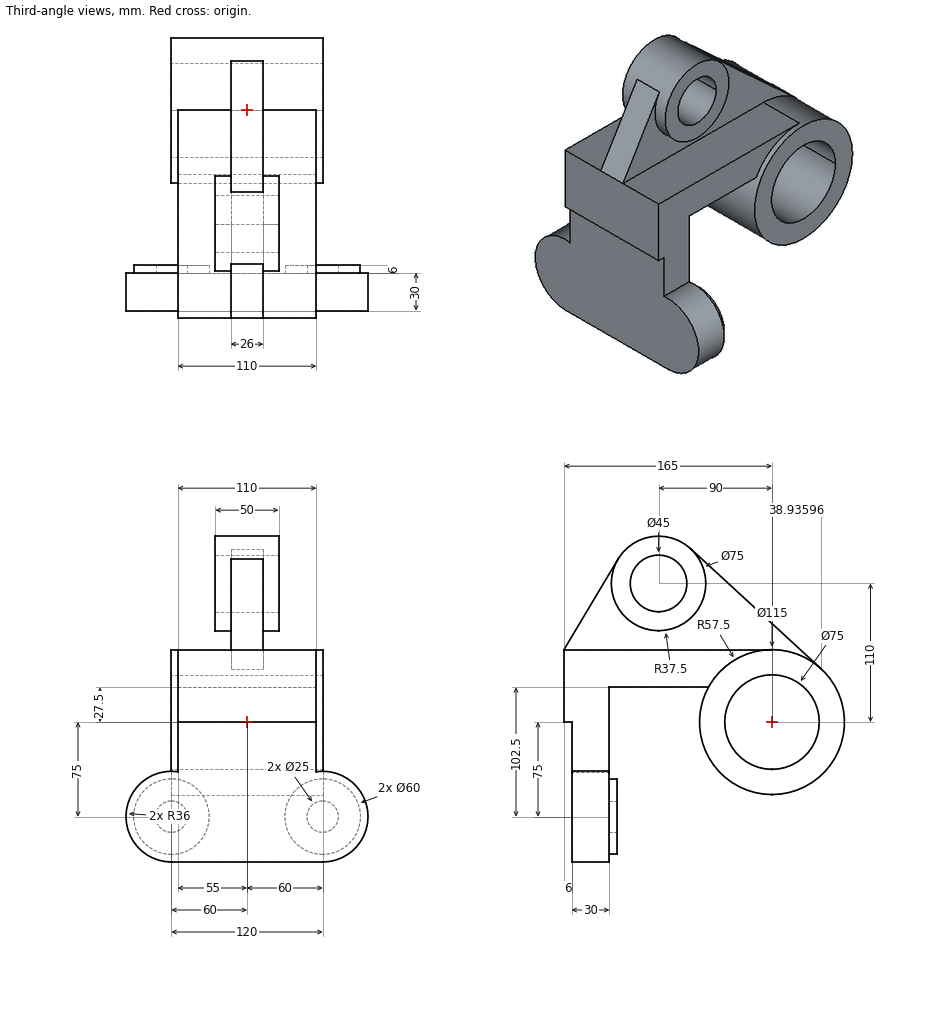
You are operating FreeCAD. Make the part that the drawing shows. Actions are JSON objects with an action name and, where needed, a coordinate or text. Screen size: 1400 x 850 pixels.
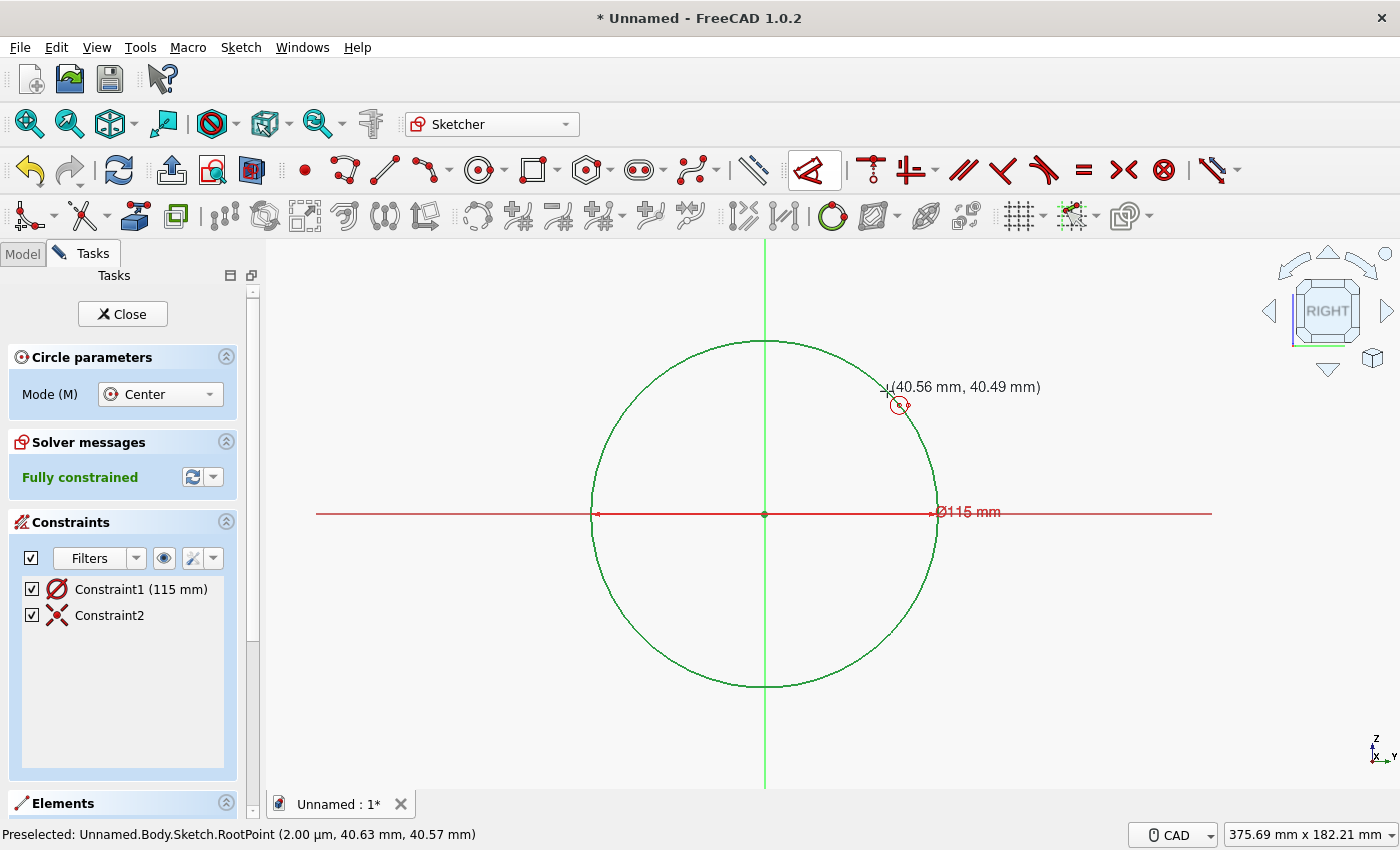
{"action": "left_click", "coordinate": [765, 514]}
{"action": "mouse_move", "coordinate": [845, 434]}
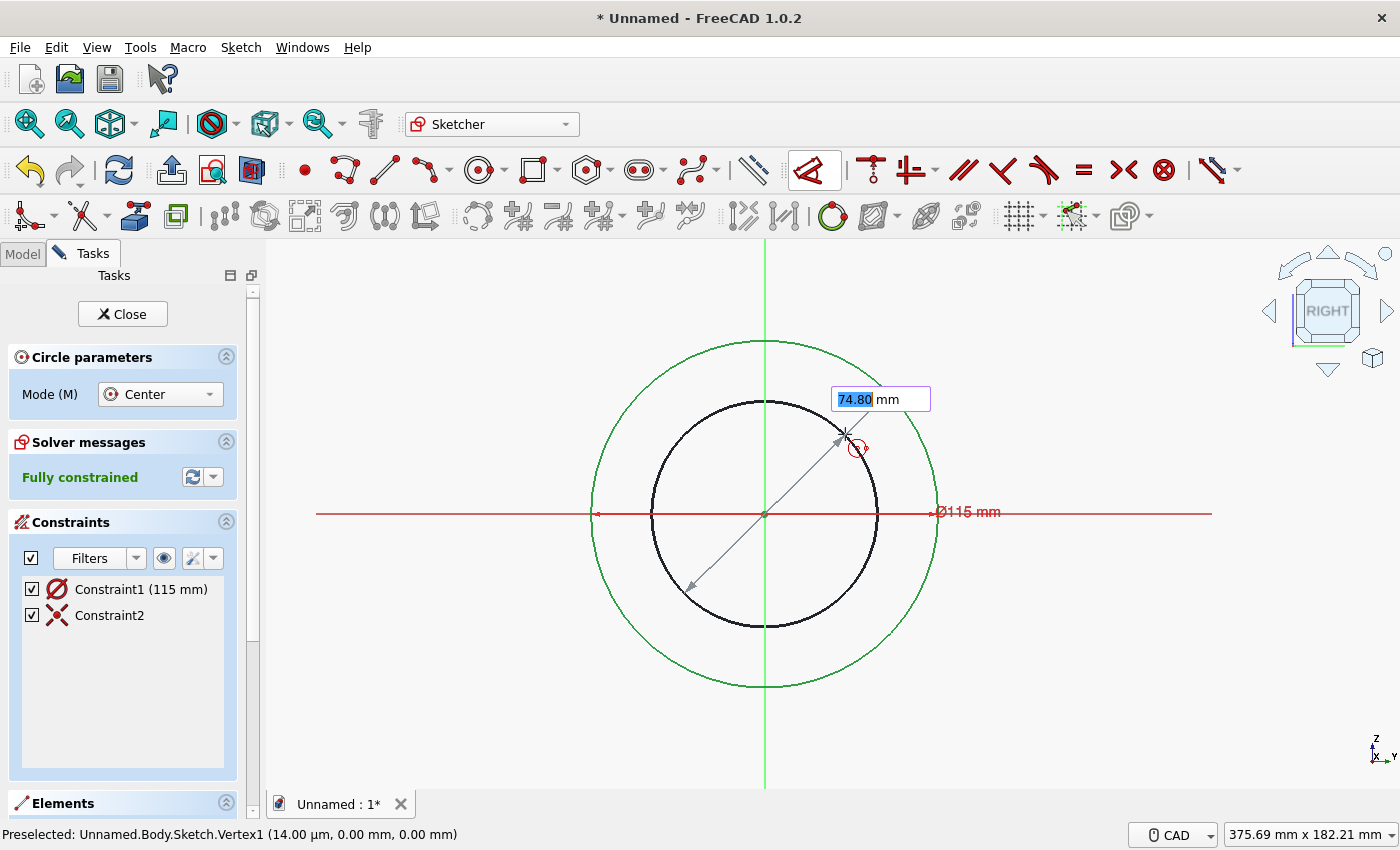
{"action": "type", "text": "75"}
{"action": "key", "text": "Return"}
{"action": "key", "text": "Escape"}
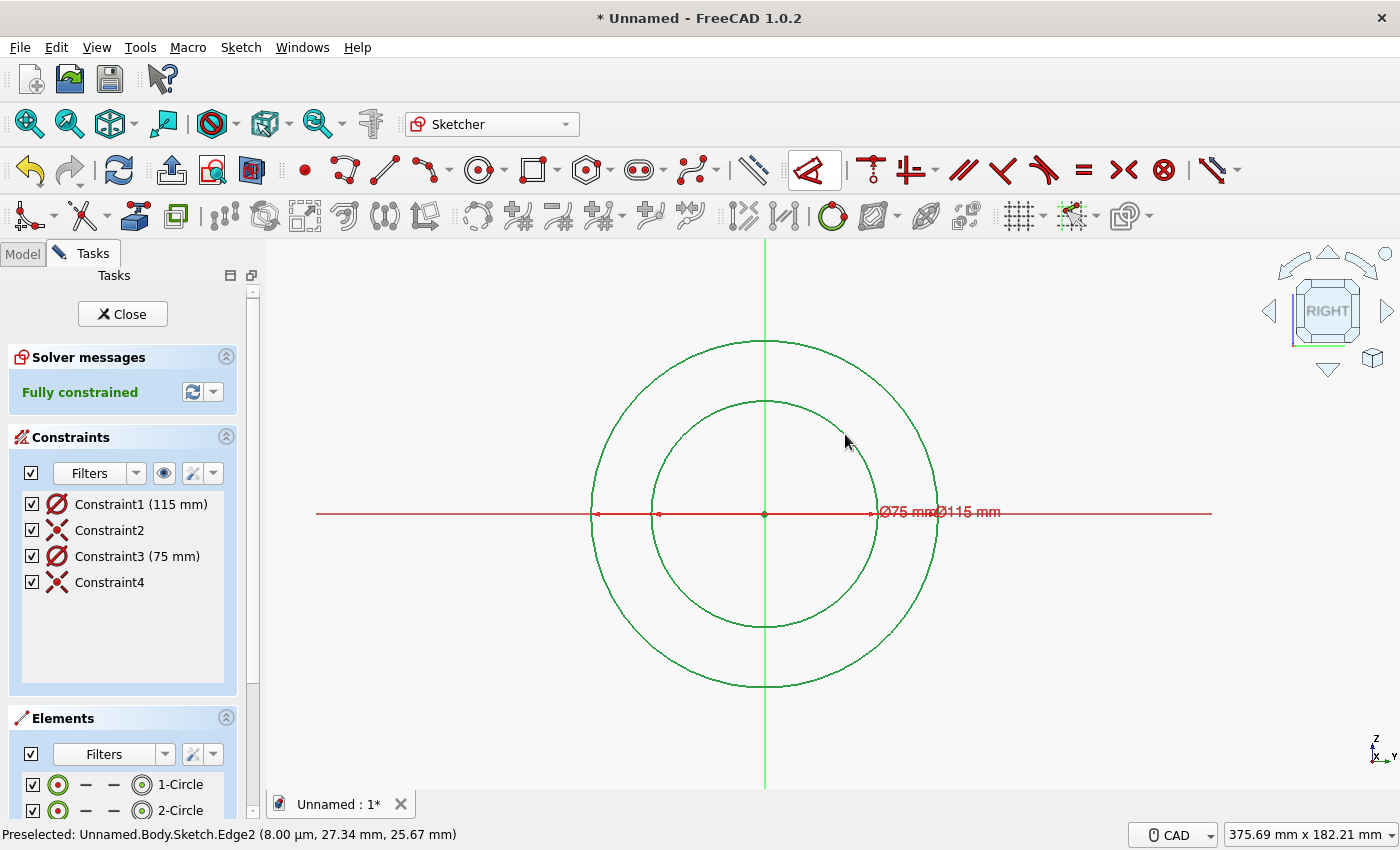
{"action": "left_click", "coordinate": [123, 314]}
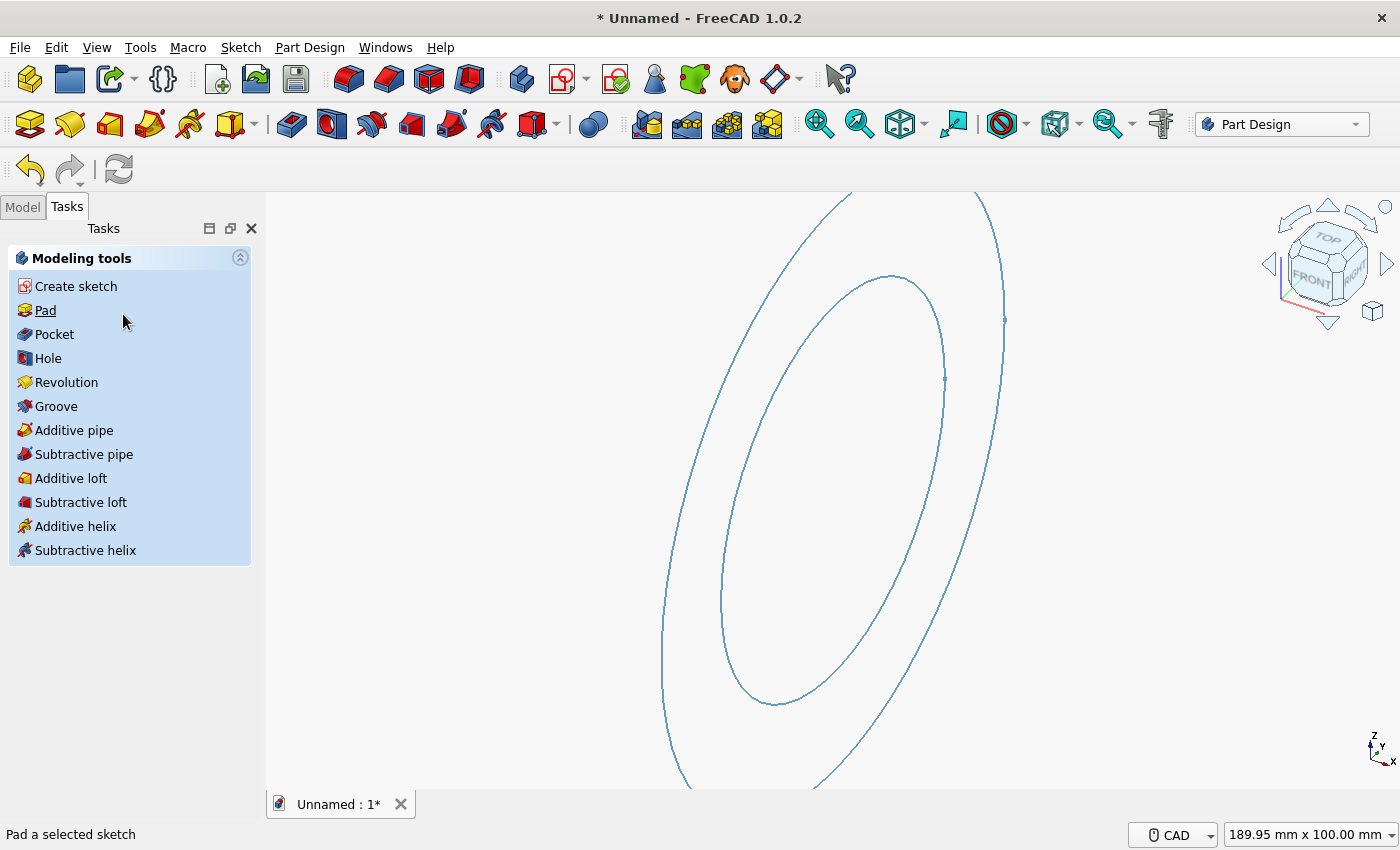
{"action": "left_click", "coordinate": [30, 124]}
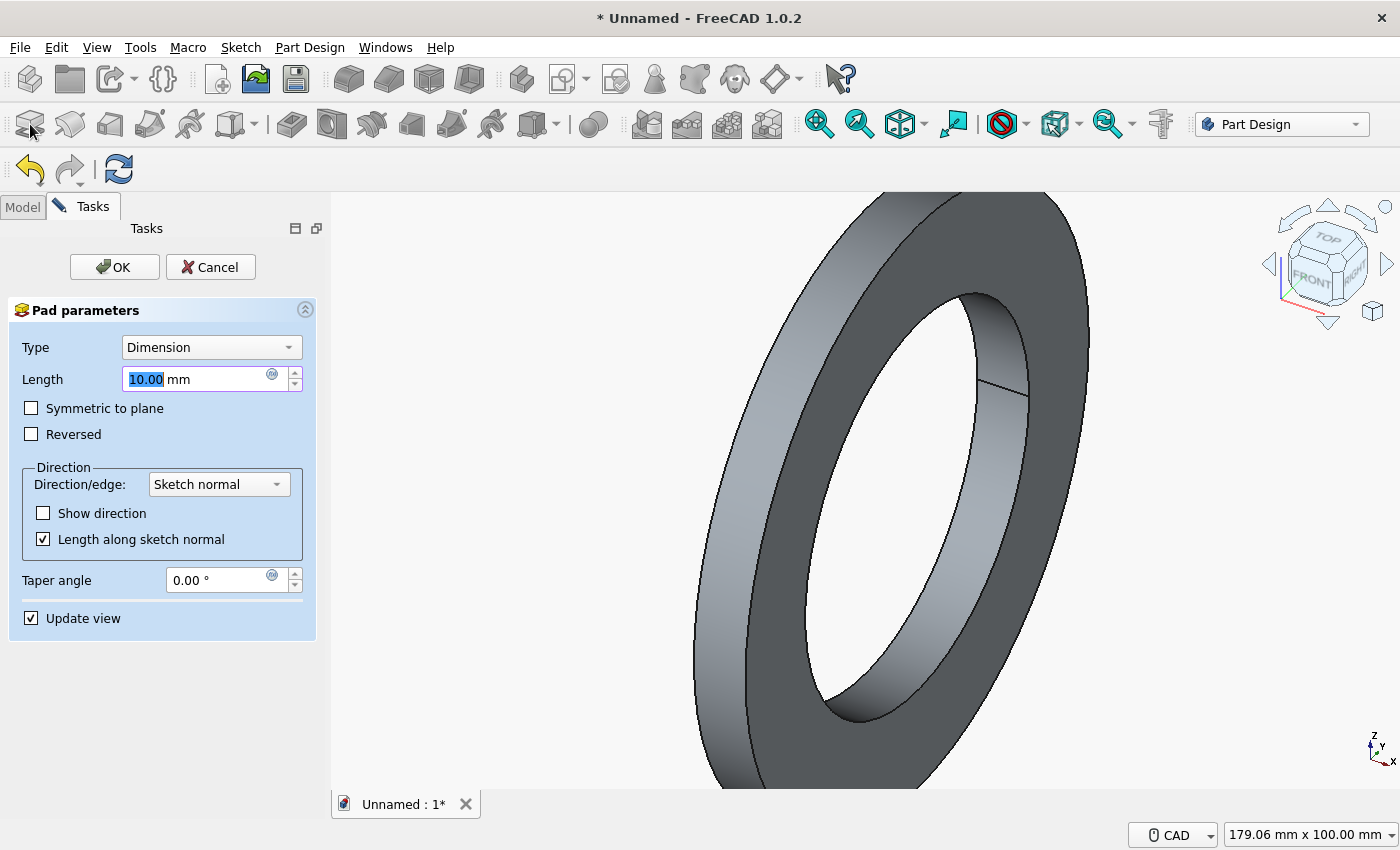
{"action": "type", "text": "120"}
{"action": "key", "text": "Tab"}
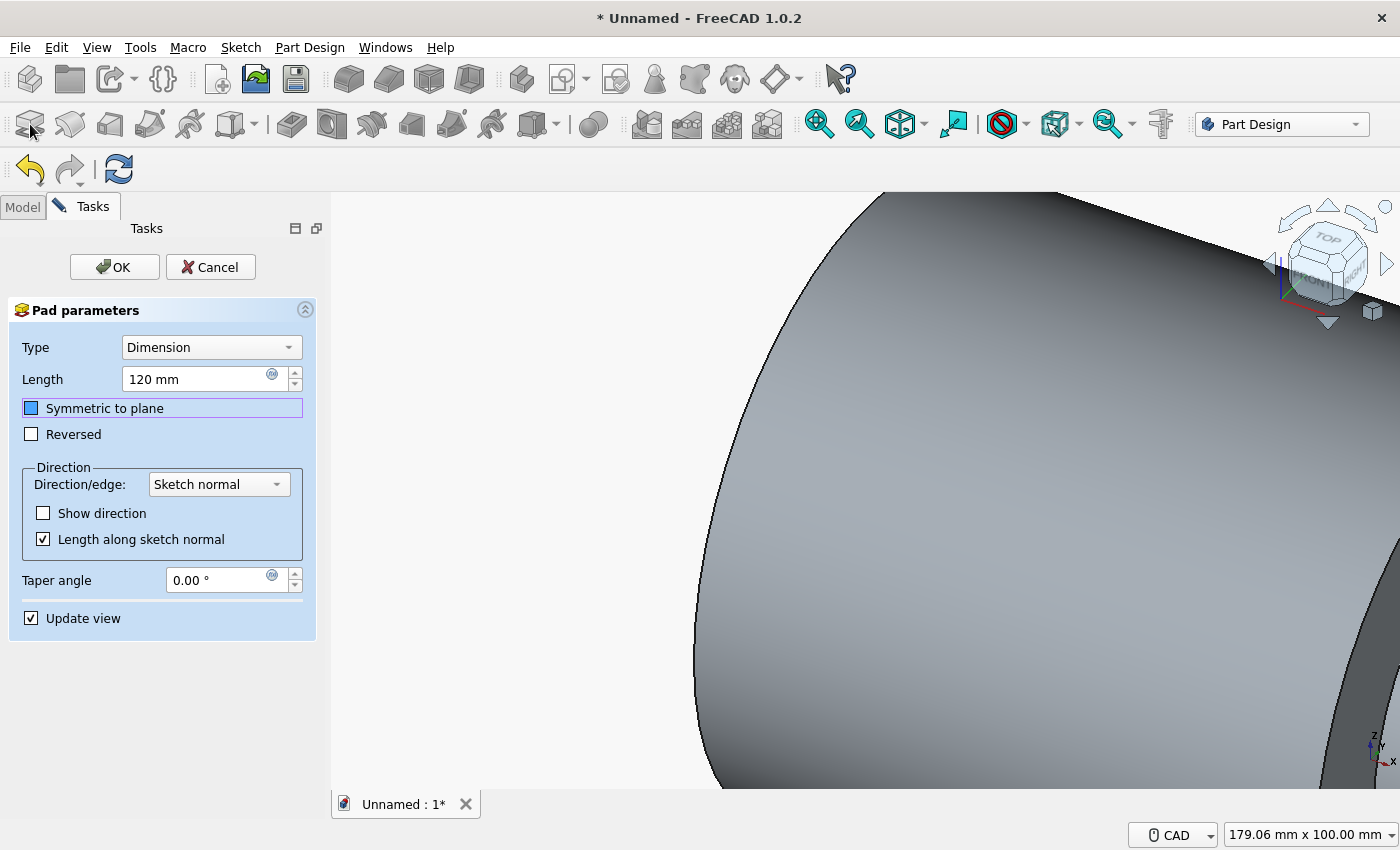
{"action": "left_click", "coordinate": [30, 408]}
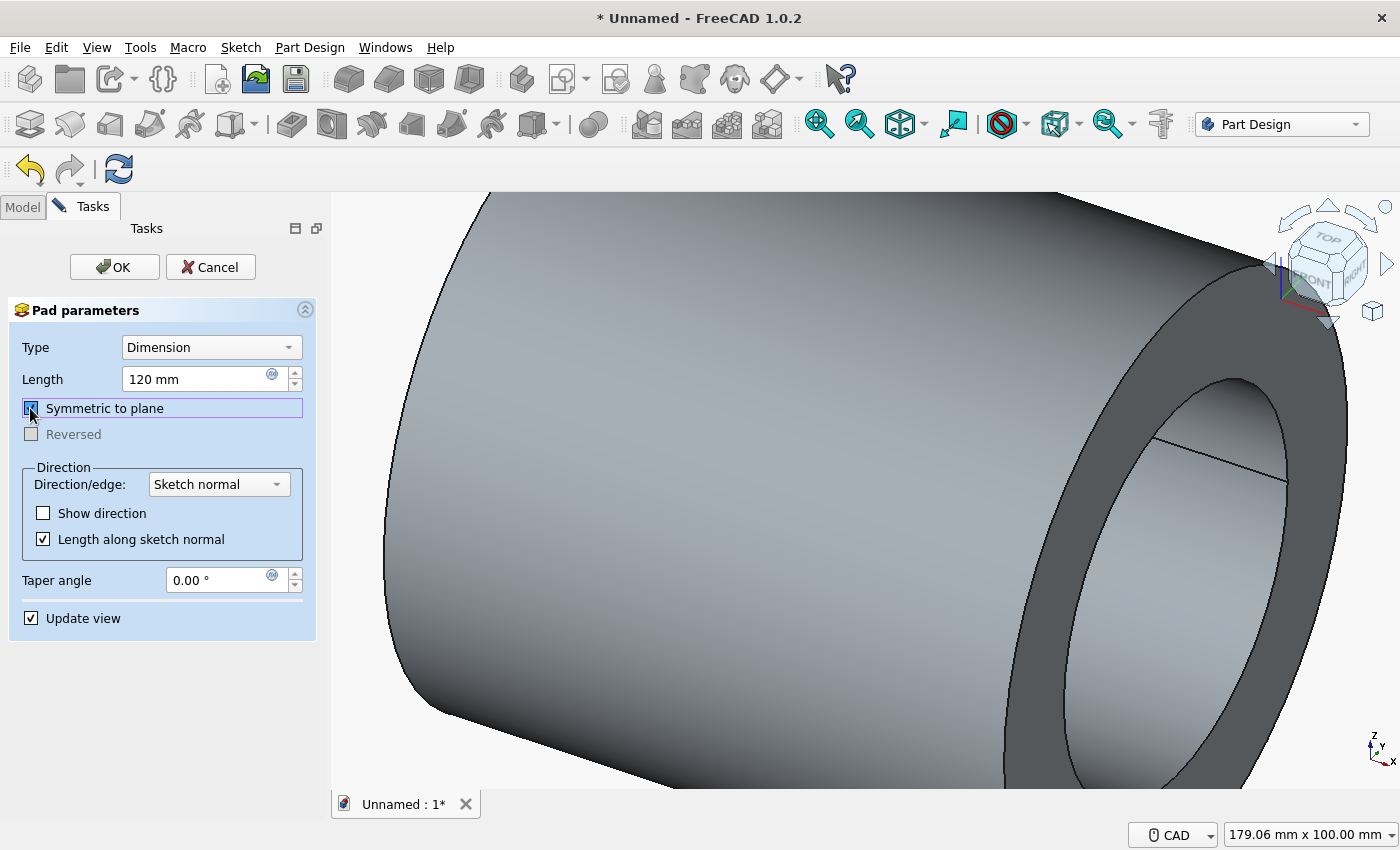
{"action": "left_click", "coordinate": [115, 267]}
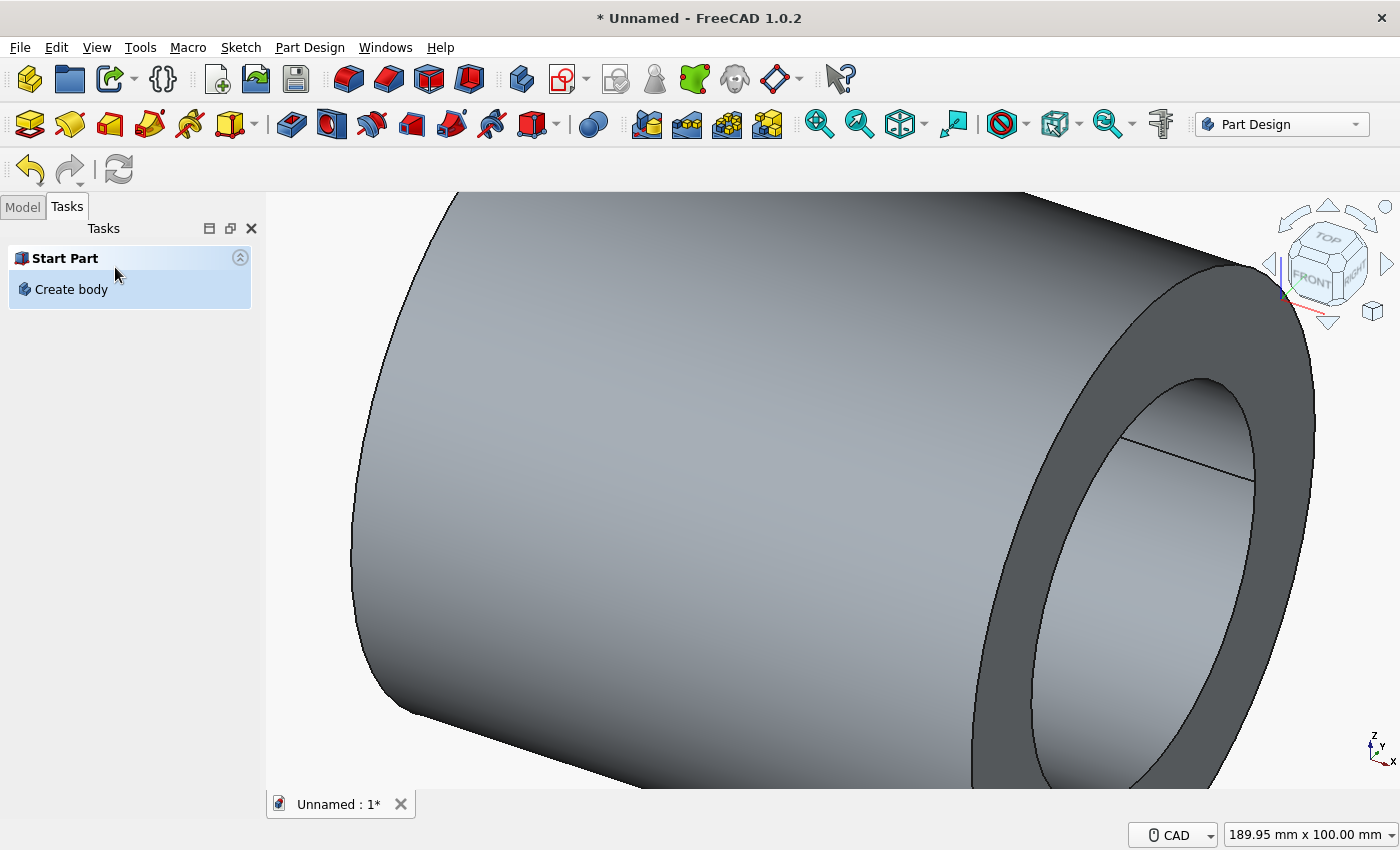
{"action": "left_click", "coordinate": [820, 124]}